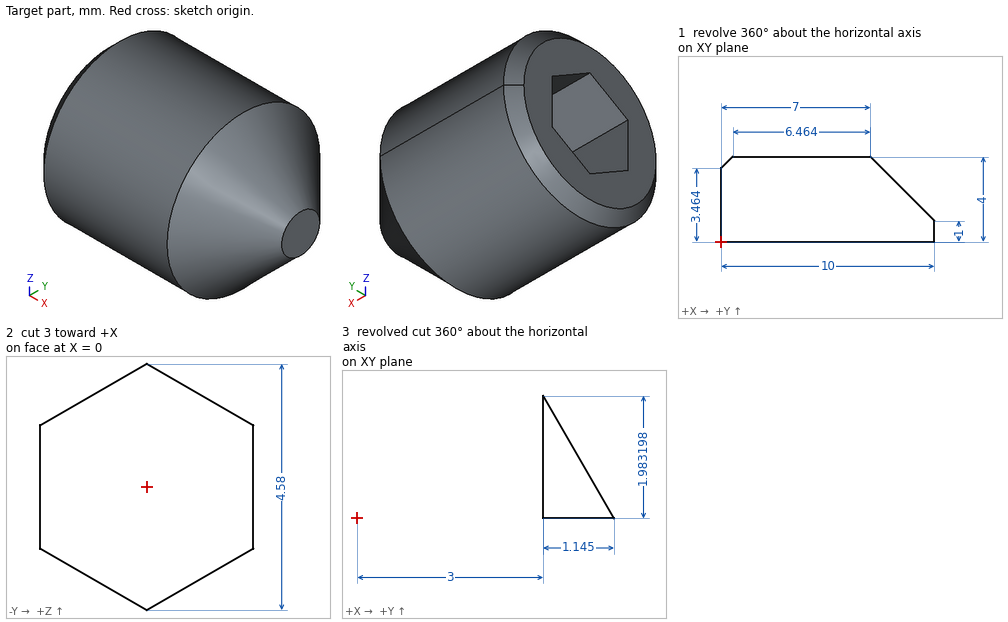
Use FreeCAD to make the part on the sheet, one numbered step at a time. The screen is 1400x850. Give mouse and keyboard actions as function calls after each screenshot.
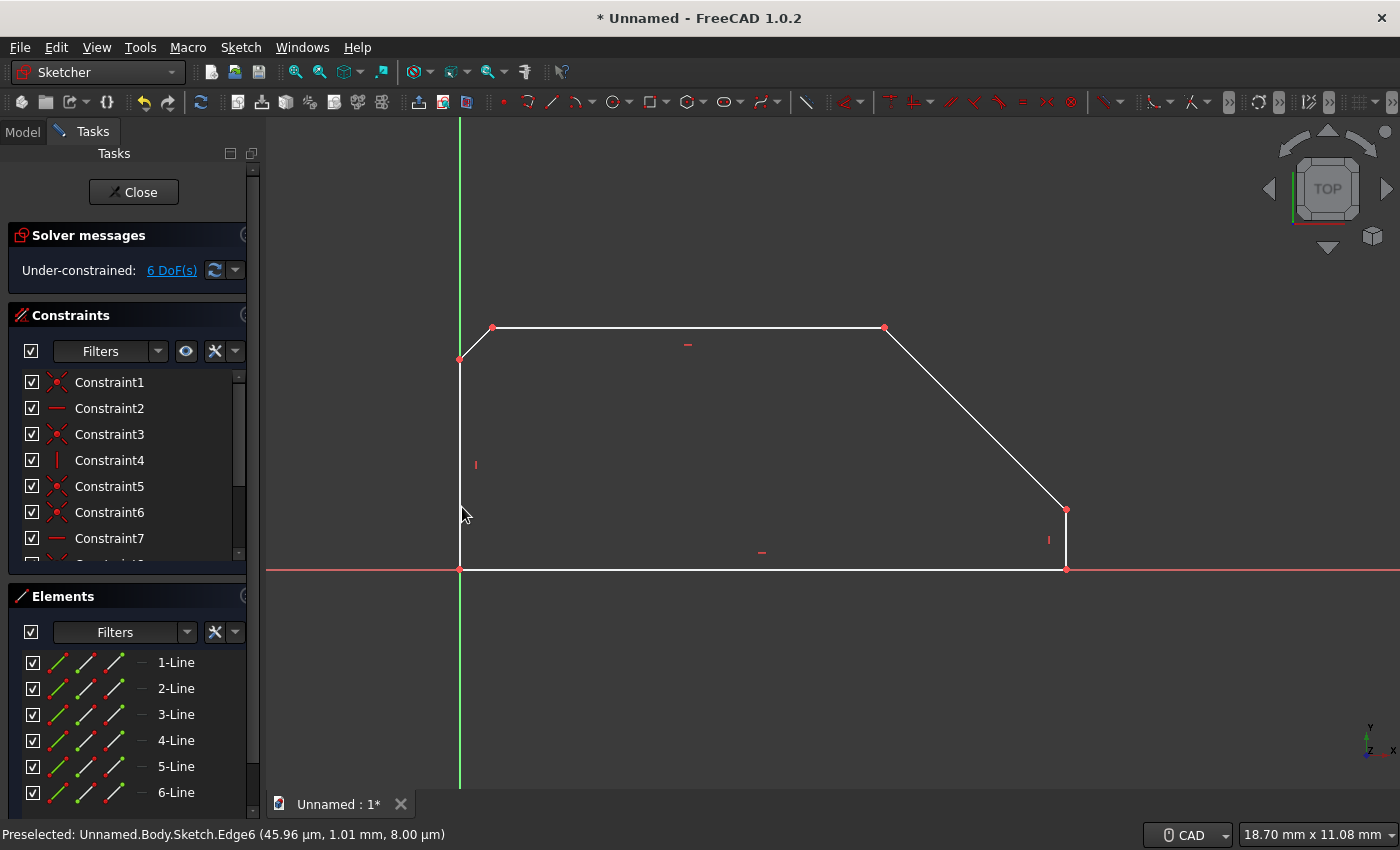
click(1066, 552)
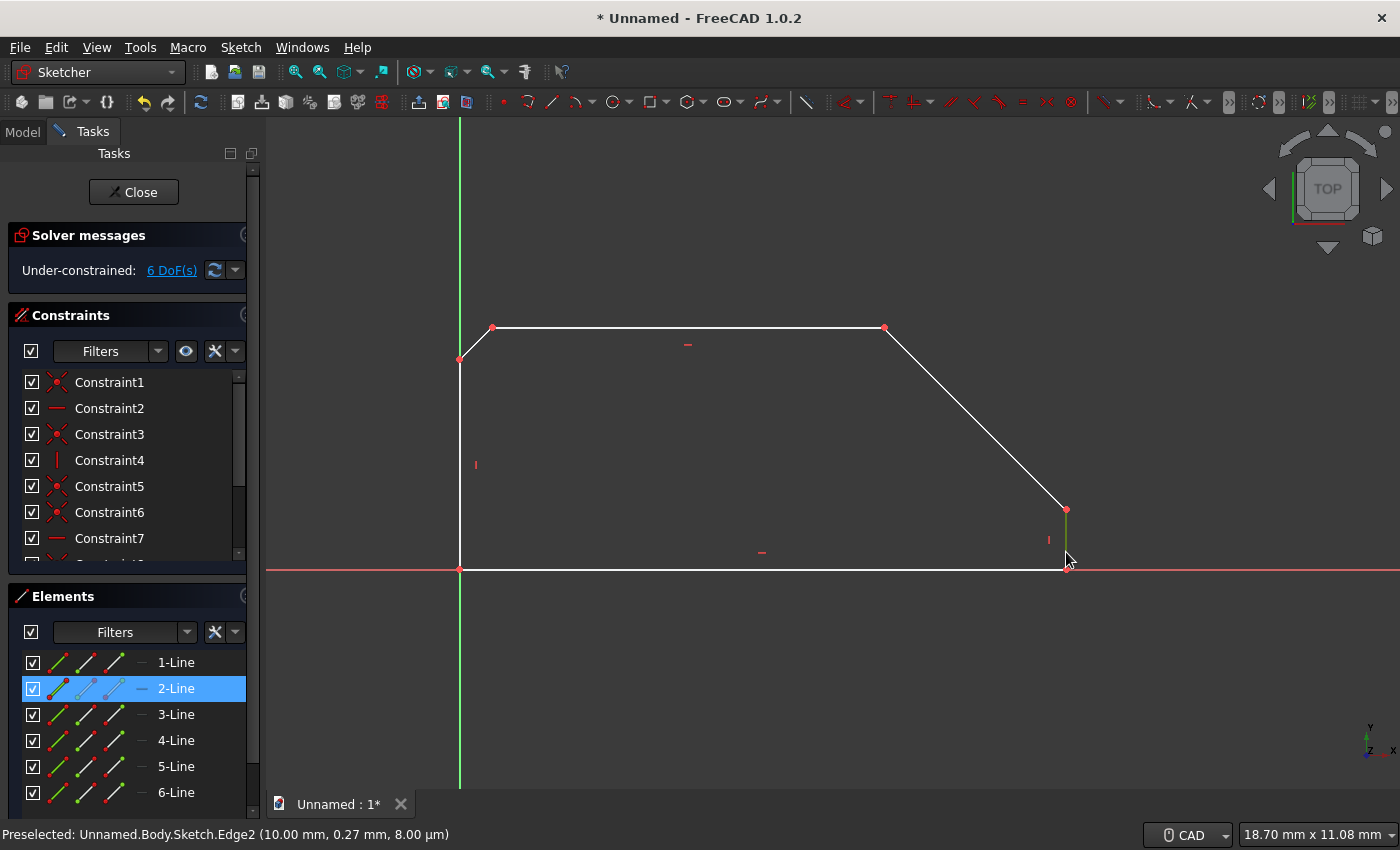
key(i)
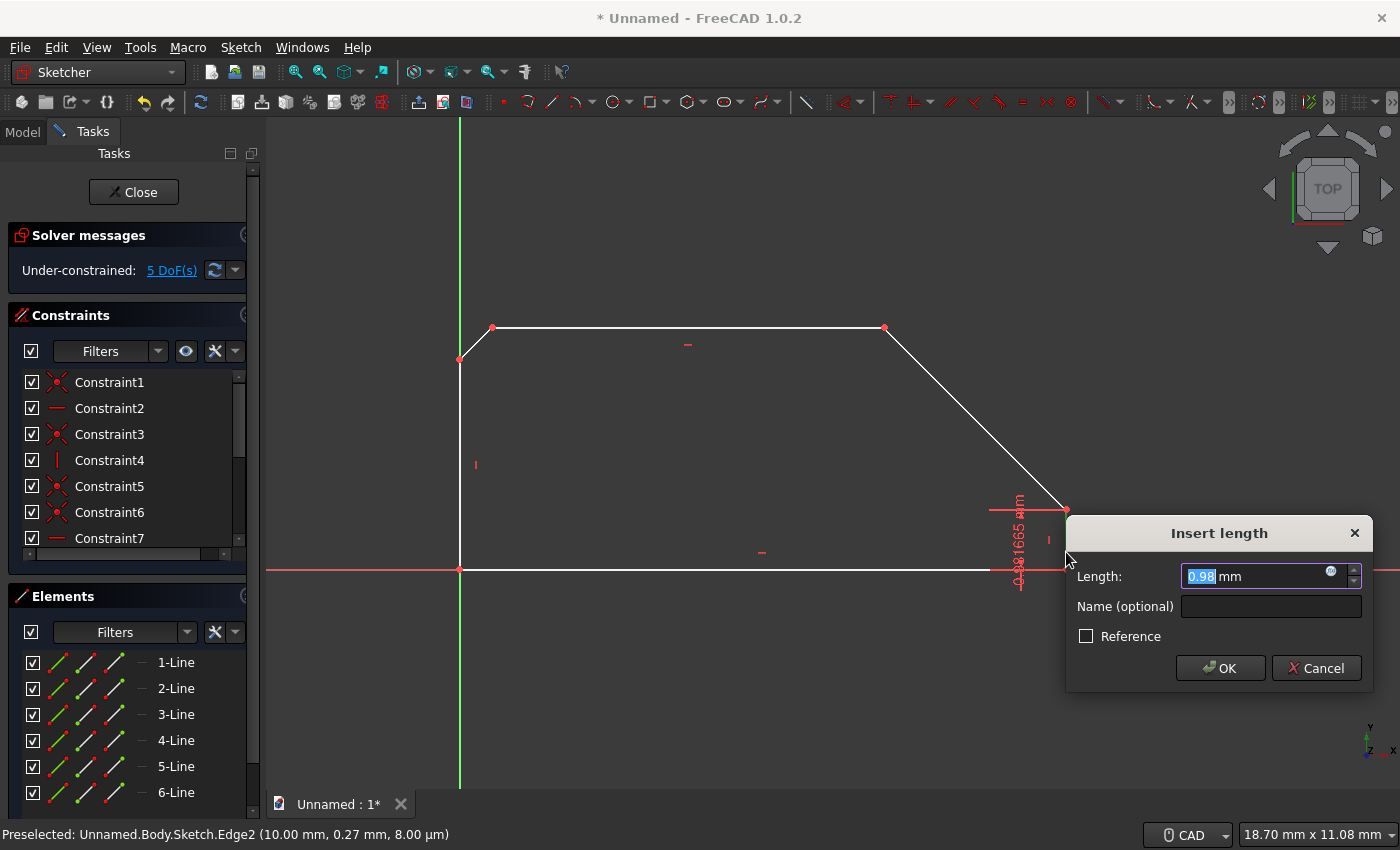
text(1)
key(Return)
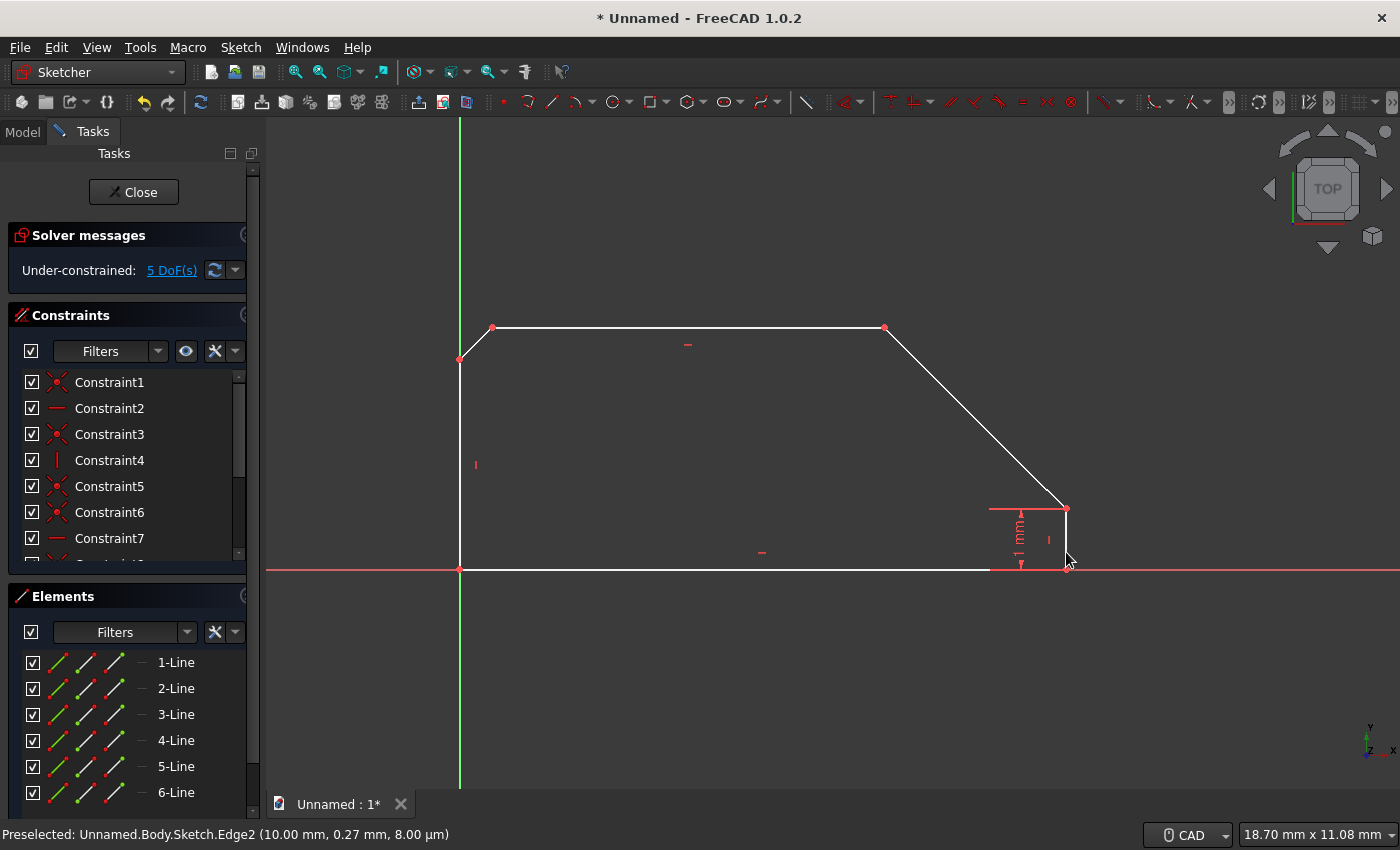
click(641, 570)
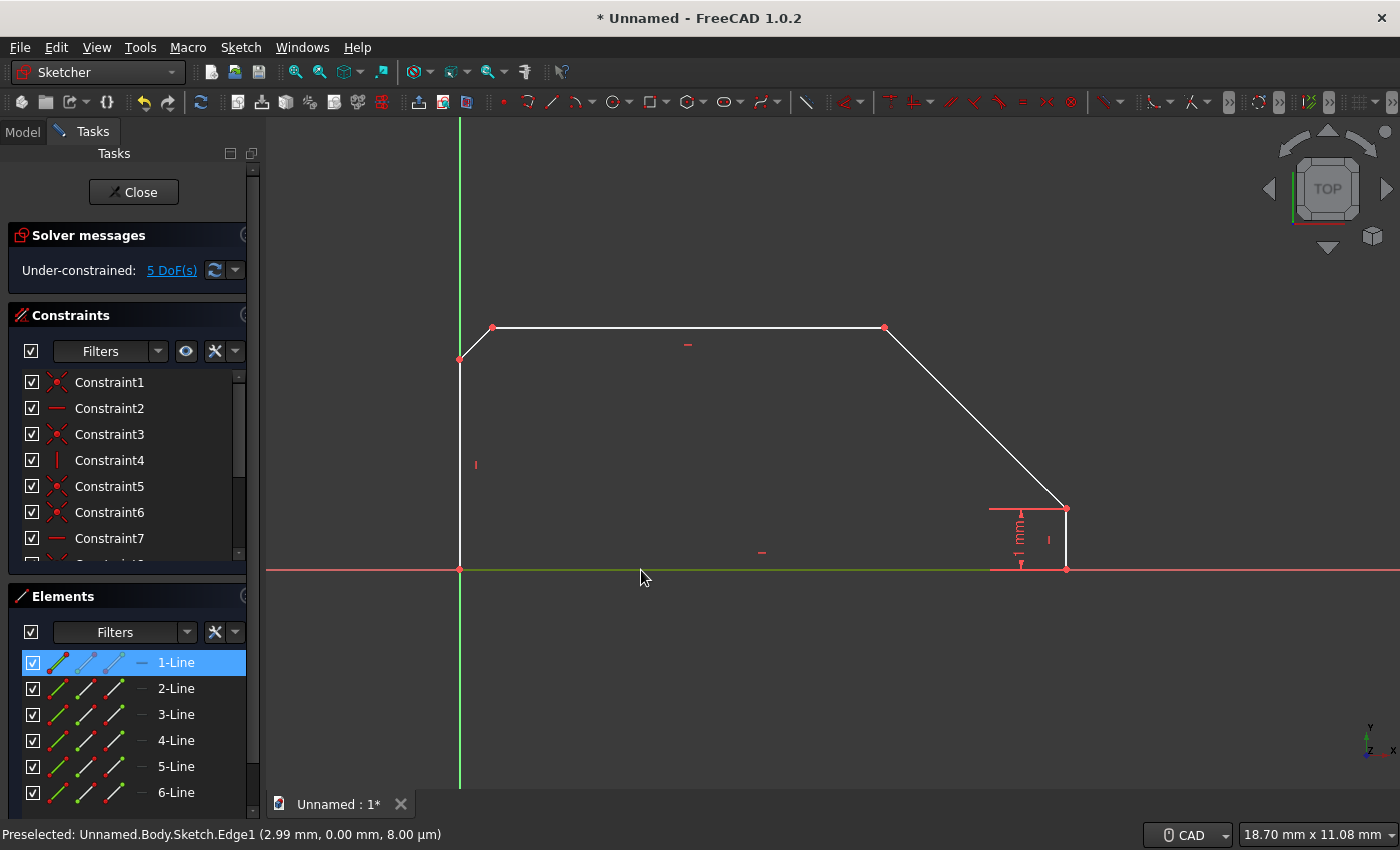
click(862, 102)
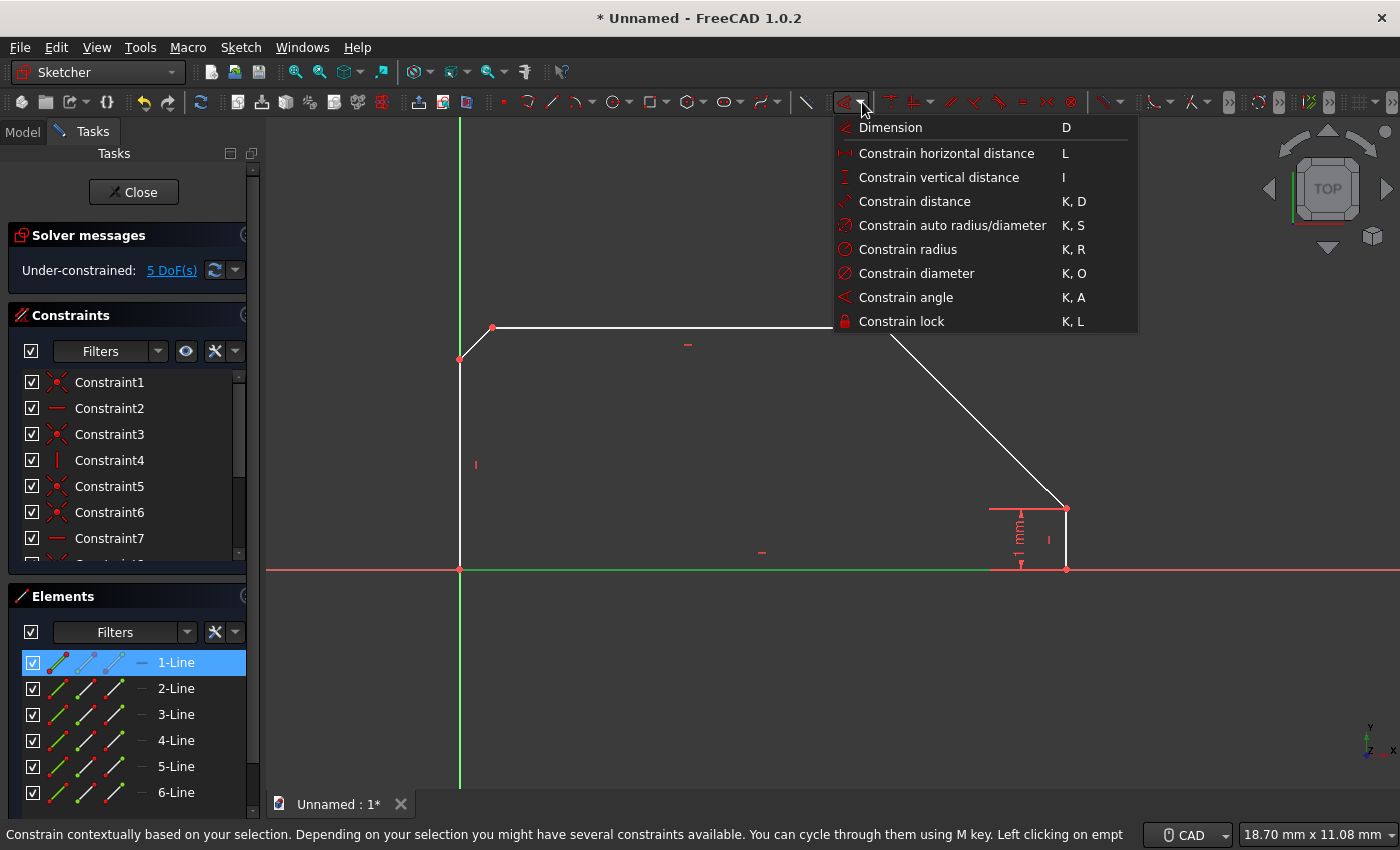
click(986, 153)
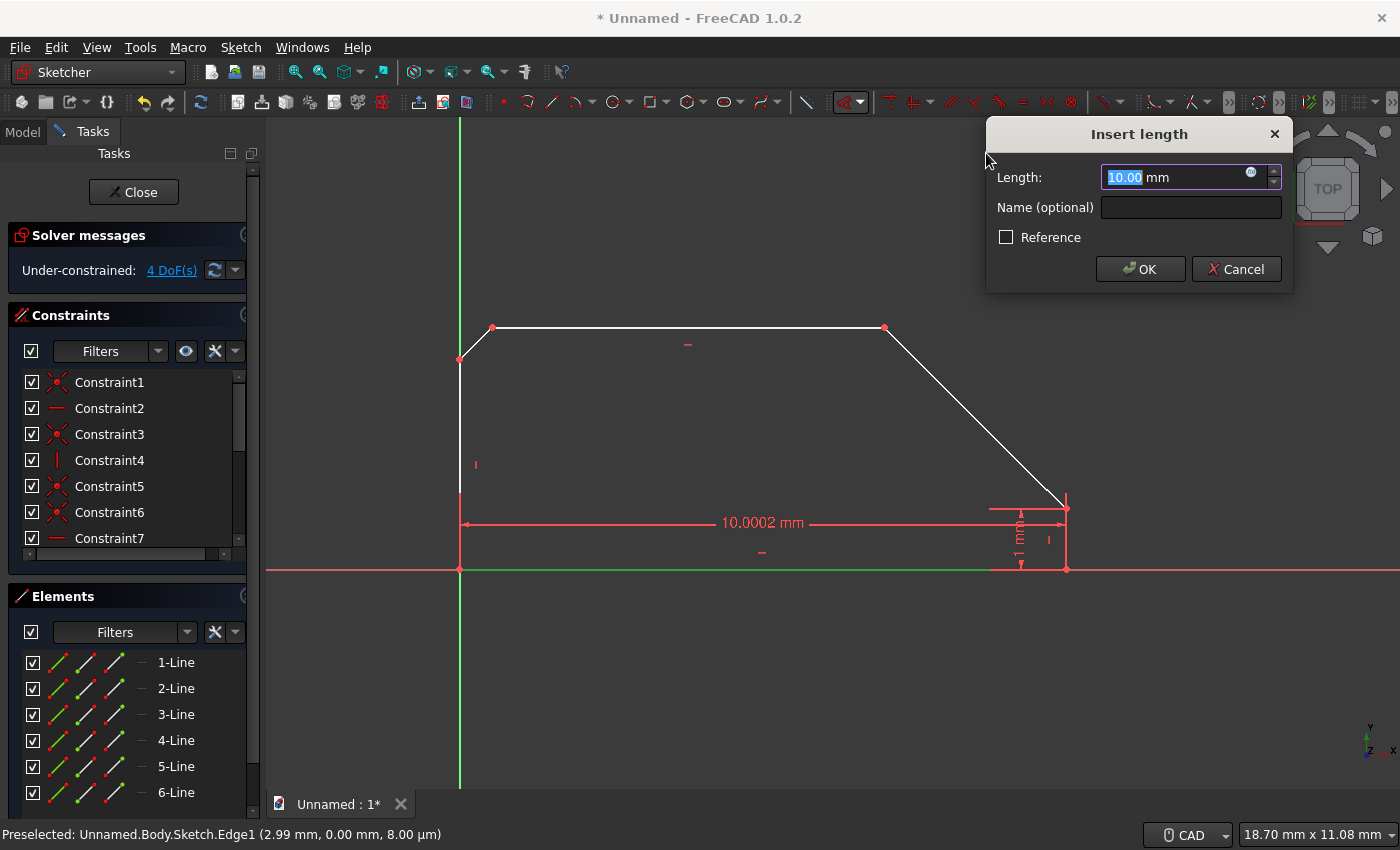
text(10)
key(Return)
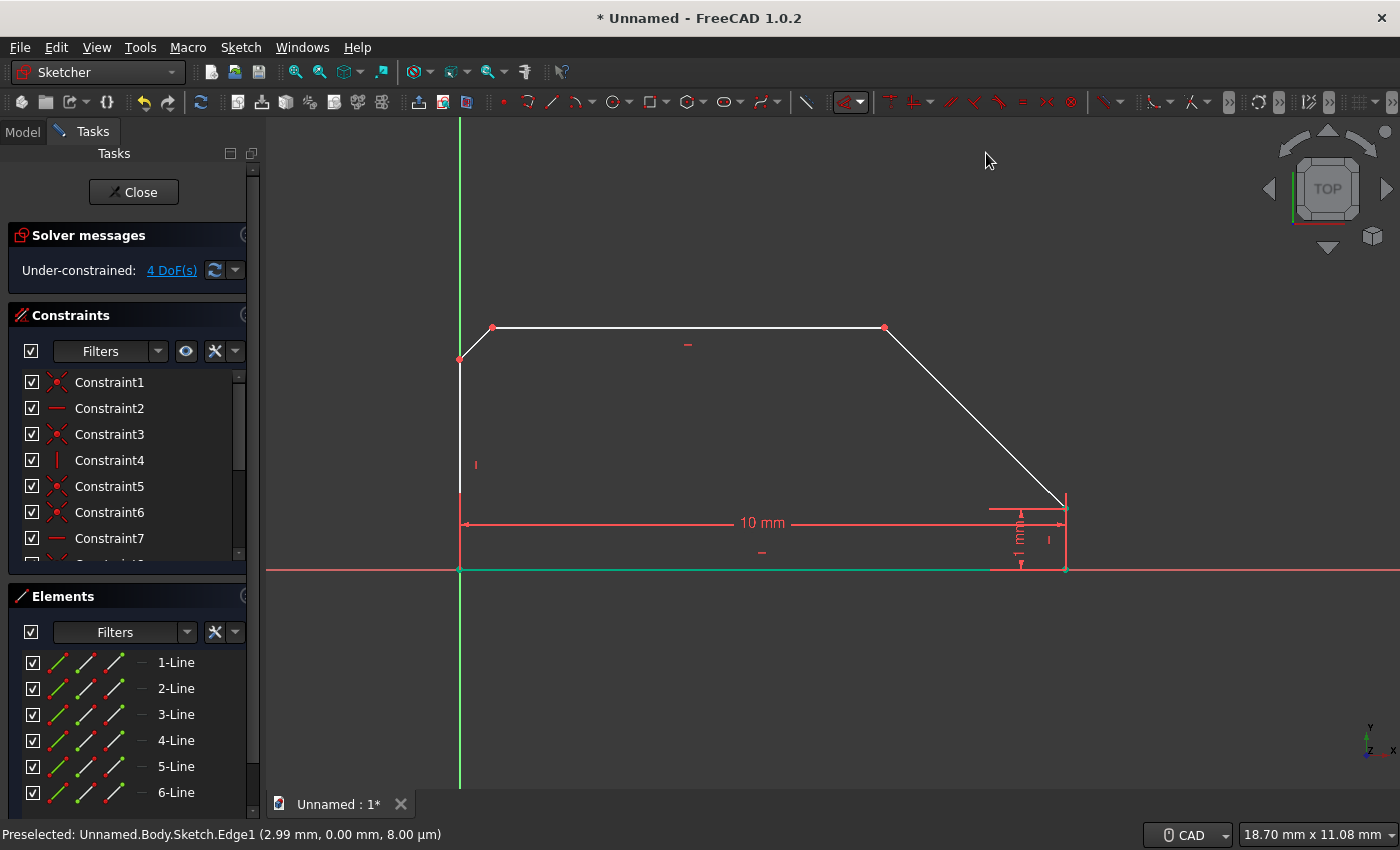
click(884, 328)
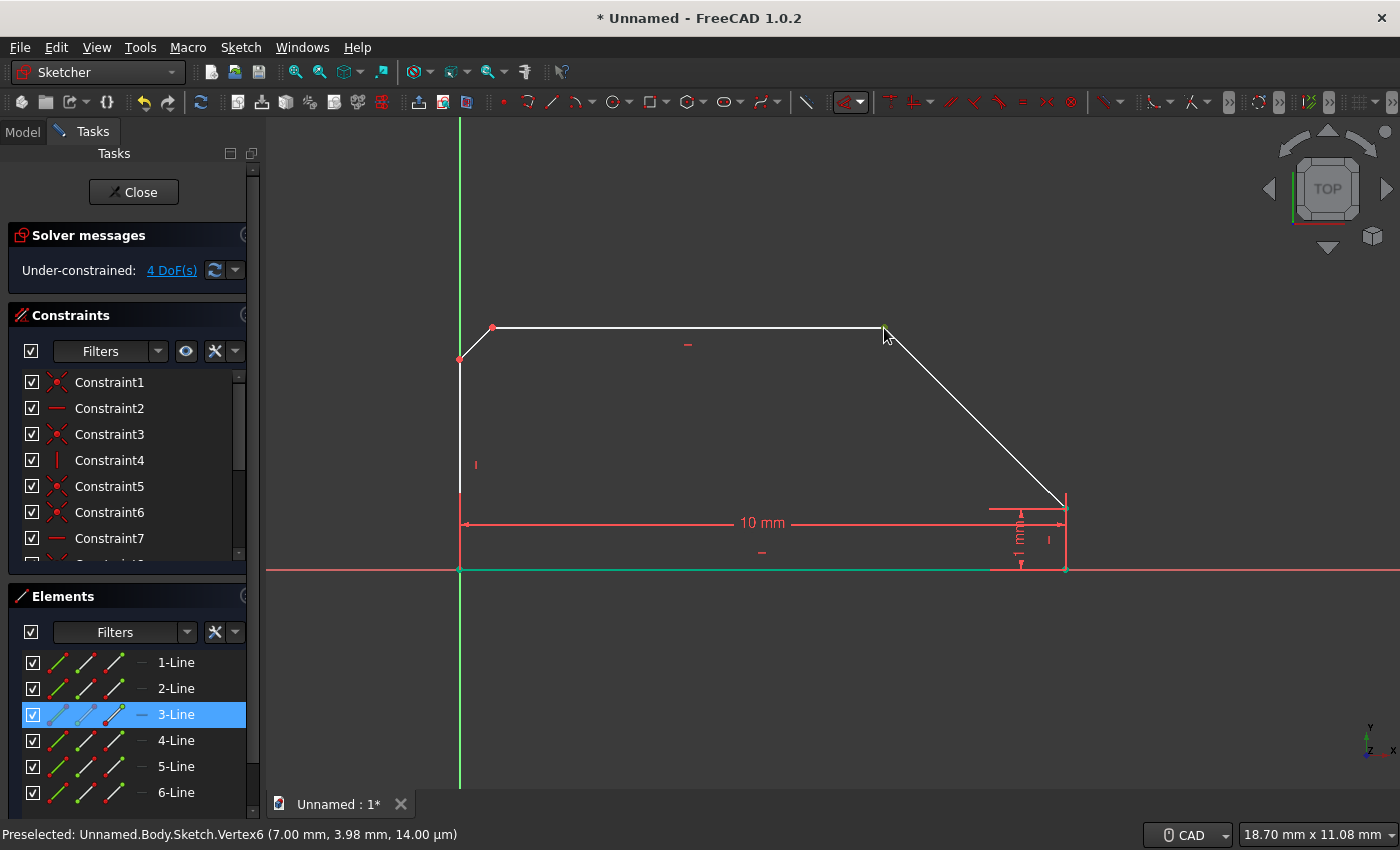
key(l)